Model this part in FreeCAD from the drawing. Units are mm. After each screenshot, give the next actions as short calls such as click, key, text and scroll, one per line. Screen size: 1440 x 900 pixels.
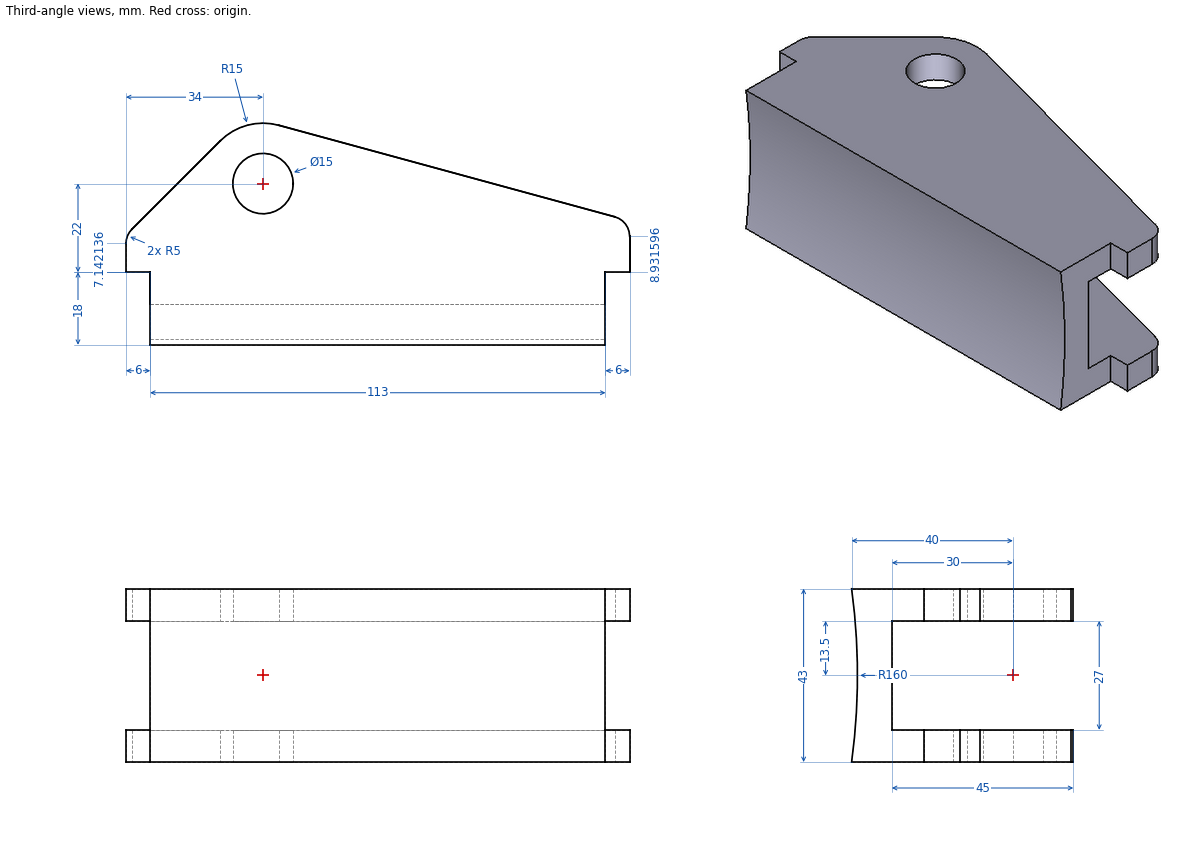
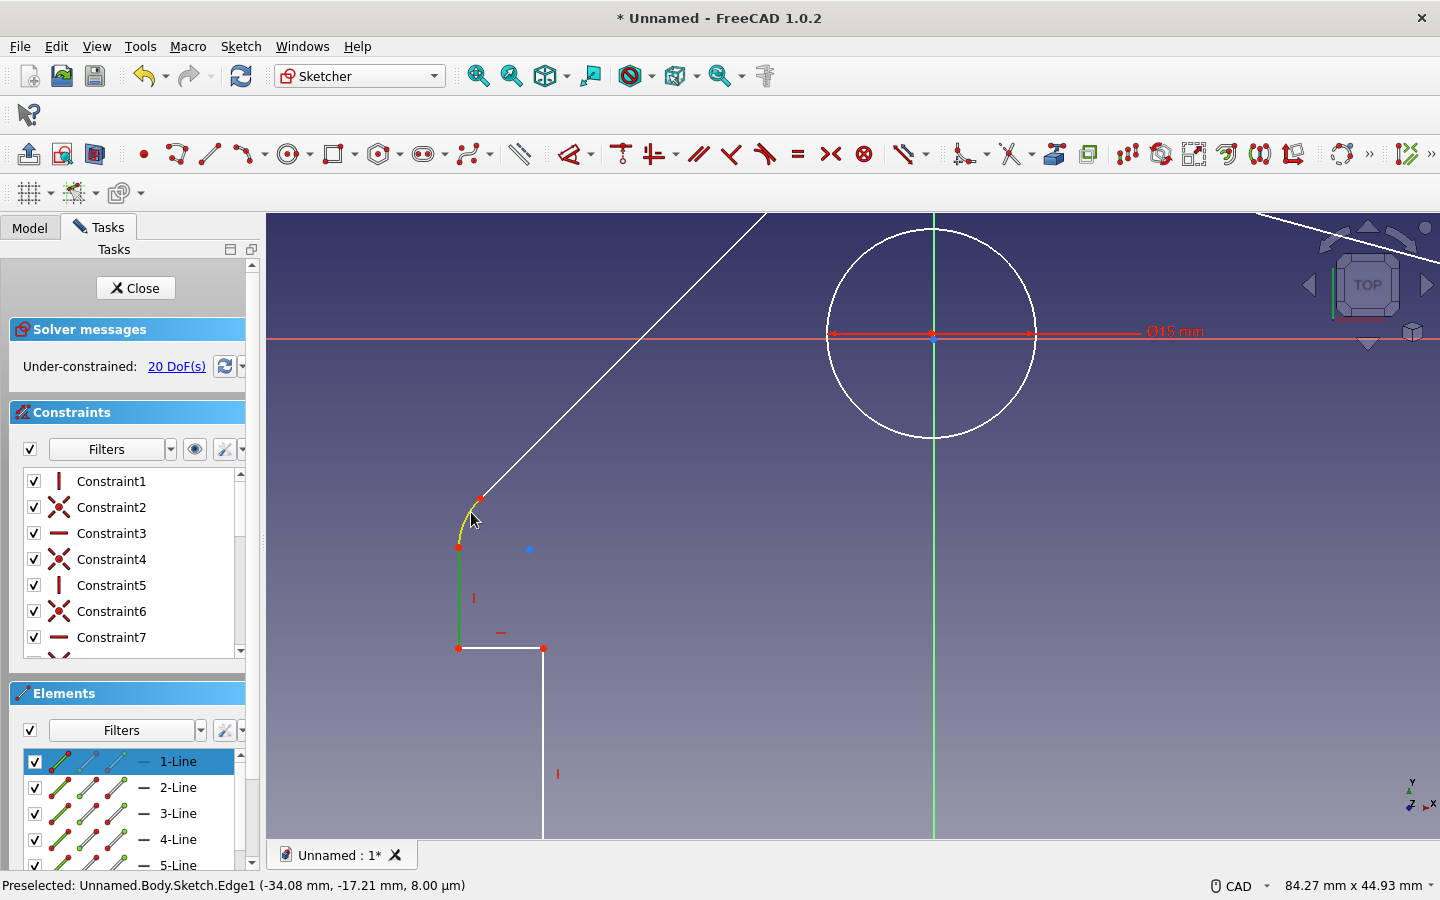
click(470, 511)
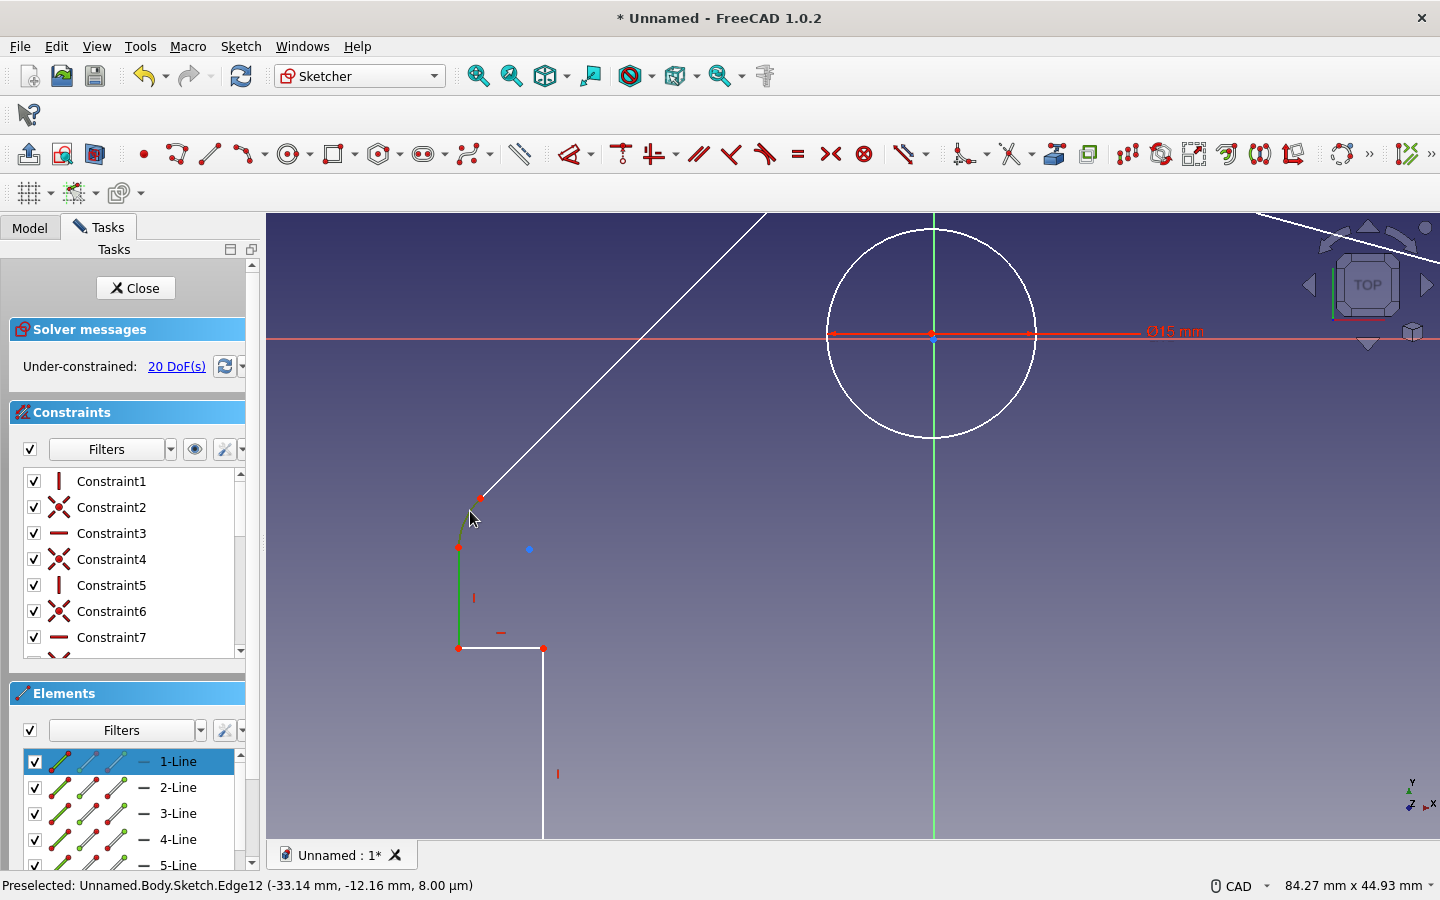
click(765, 154)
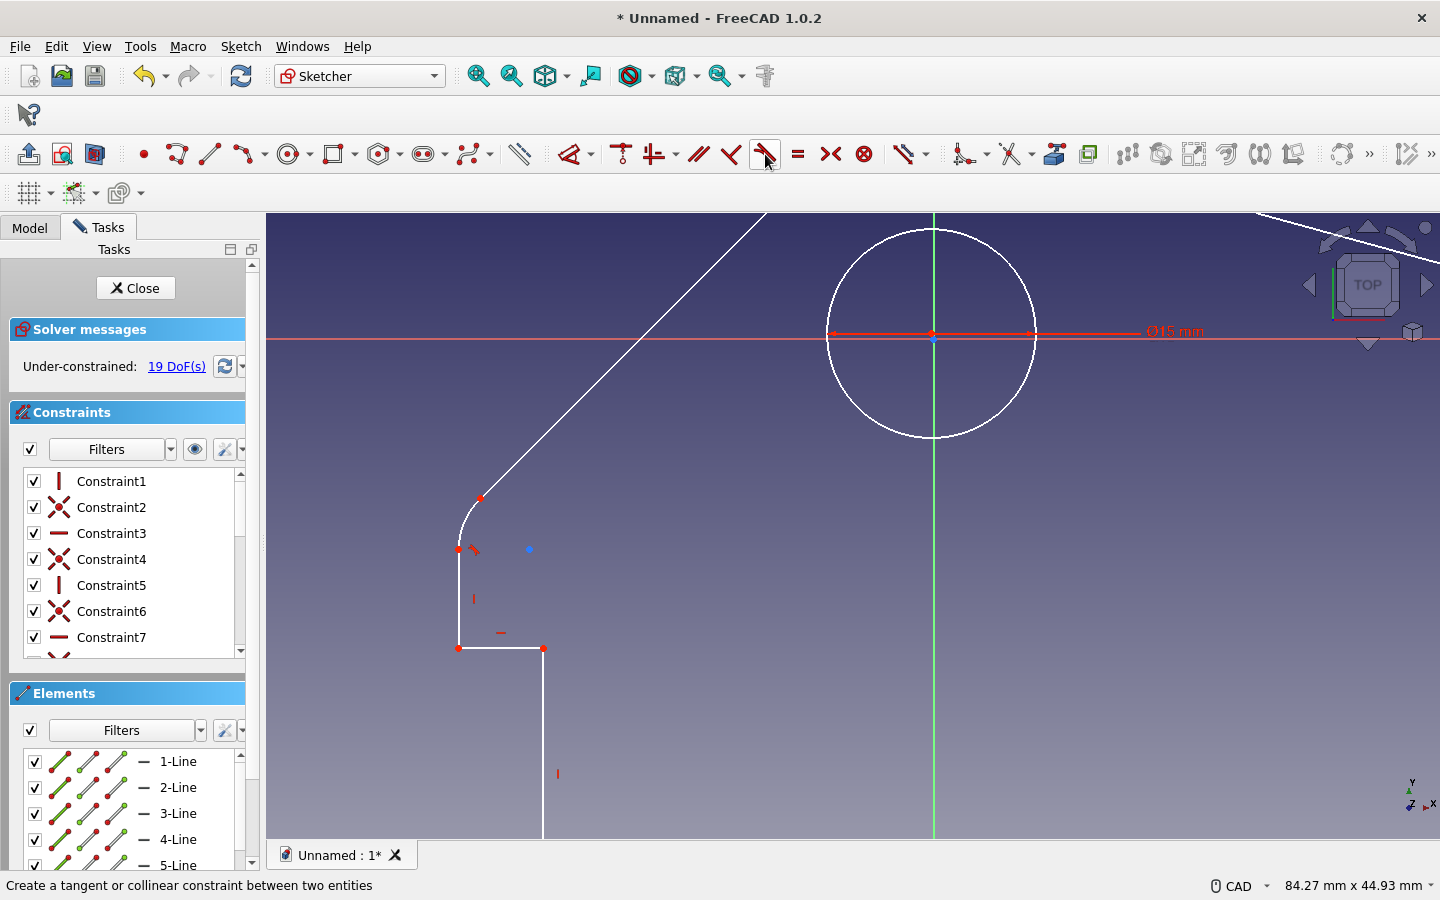
scroll(467, 531, down, 5)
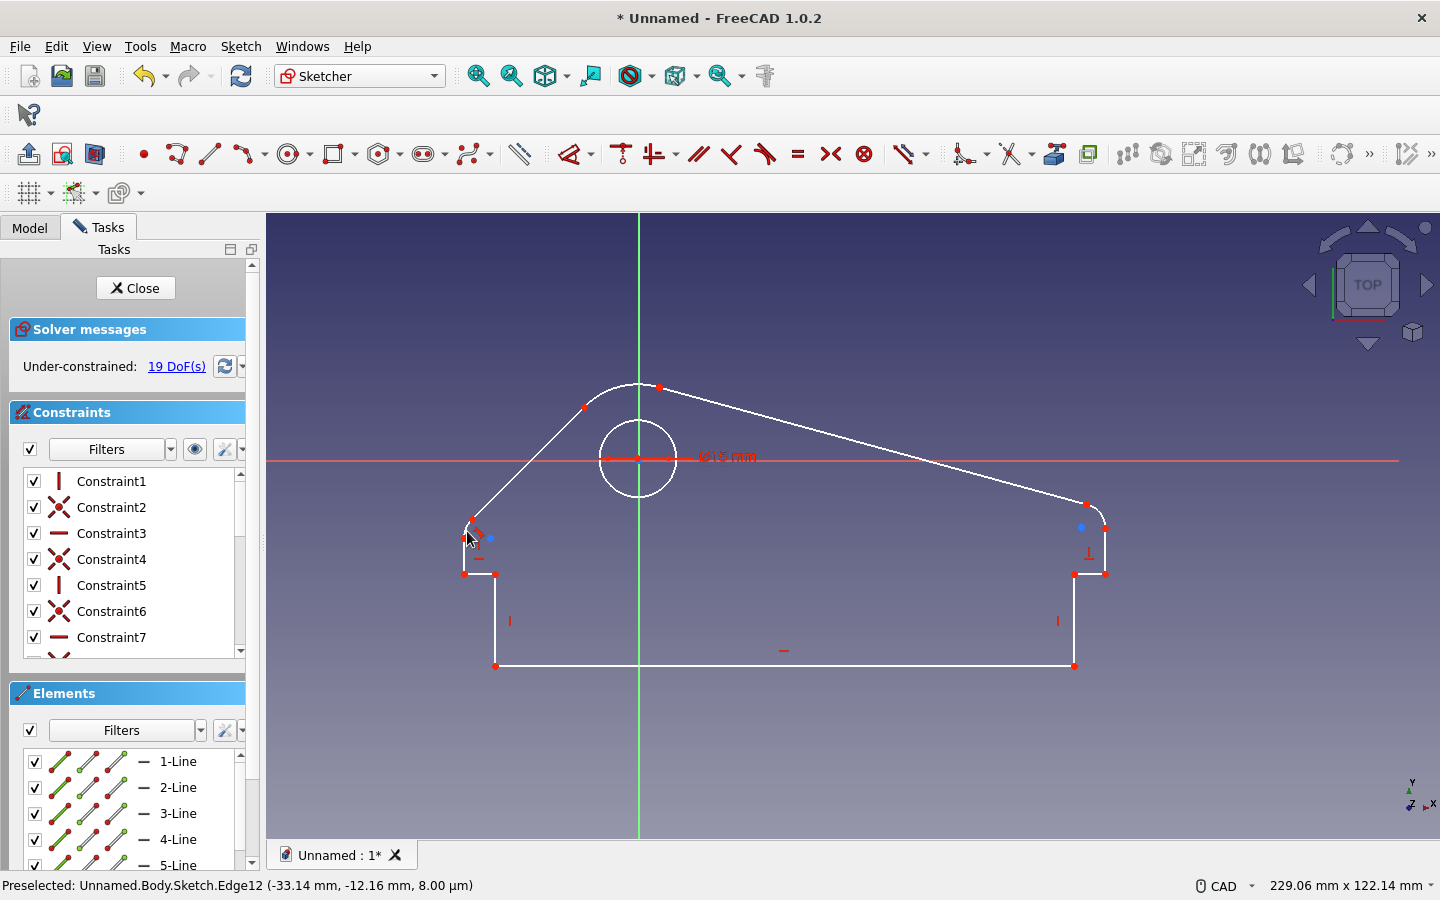
click(1105, 561)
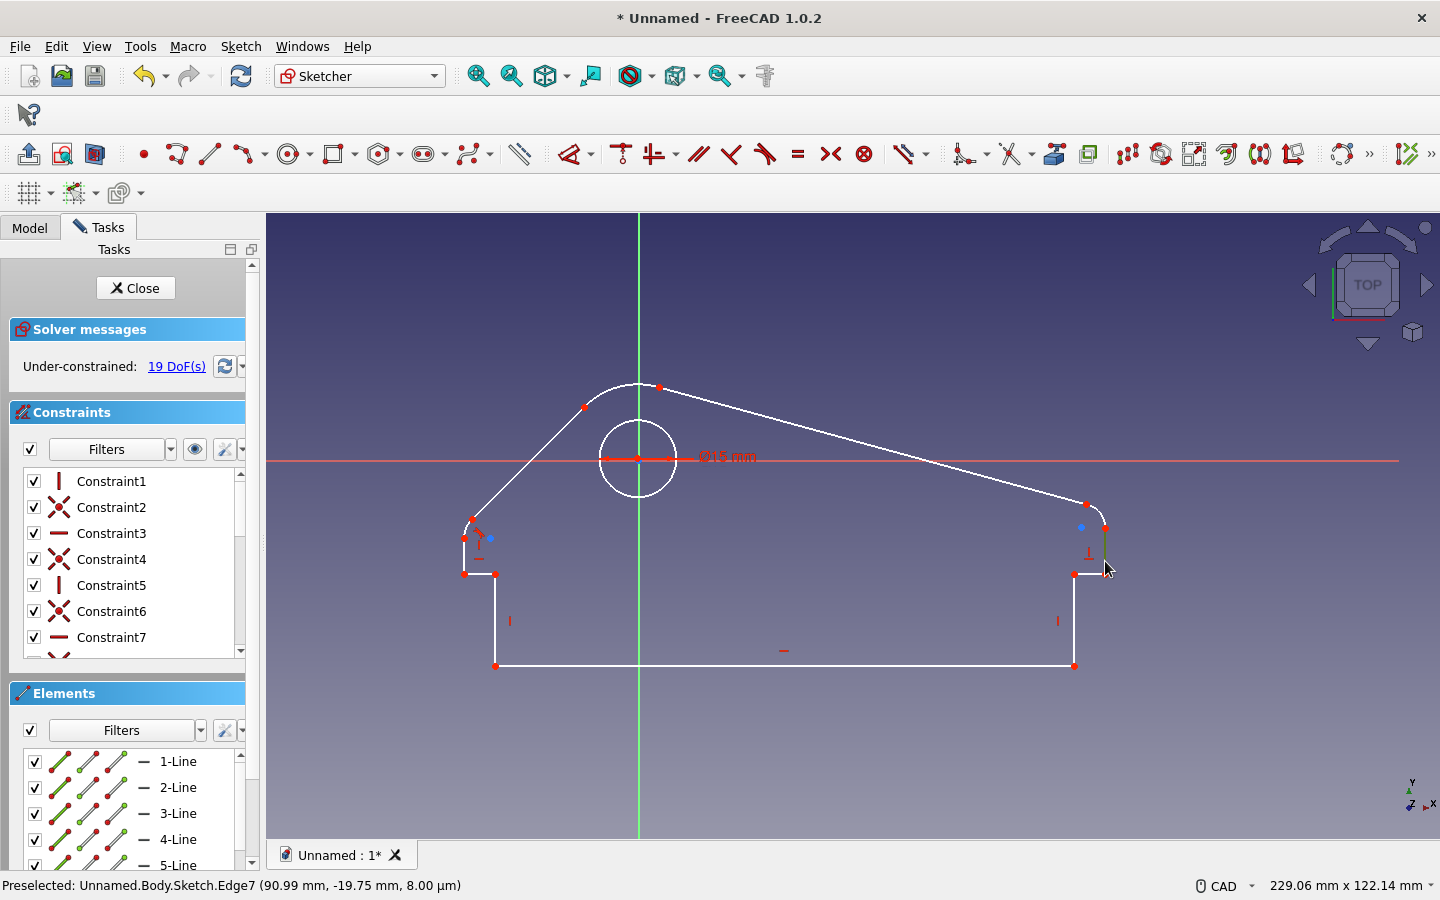
scroll(1103, 519, up, 2)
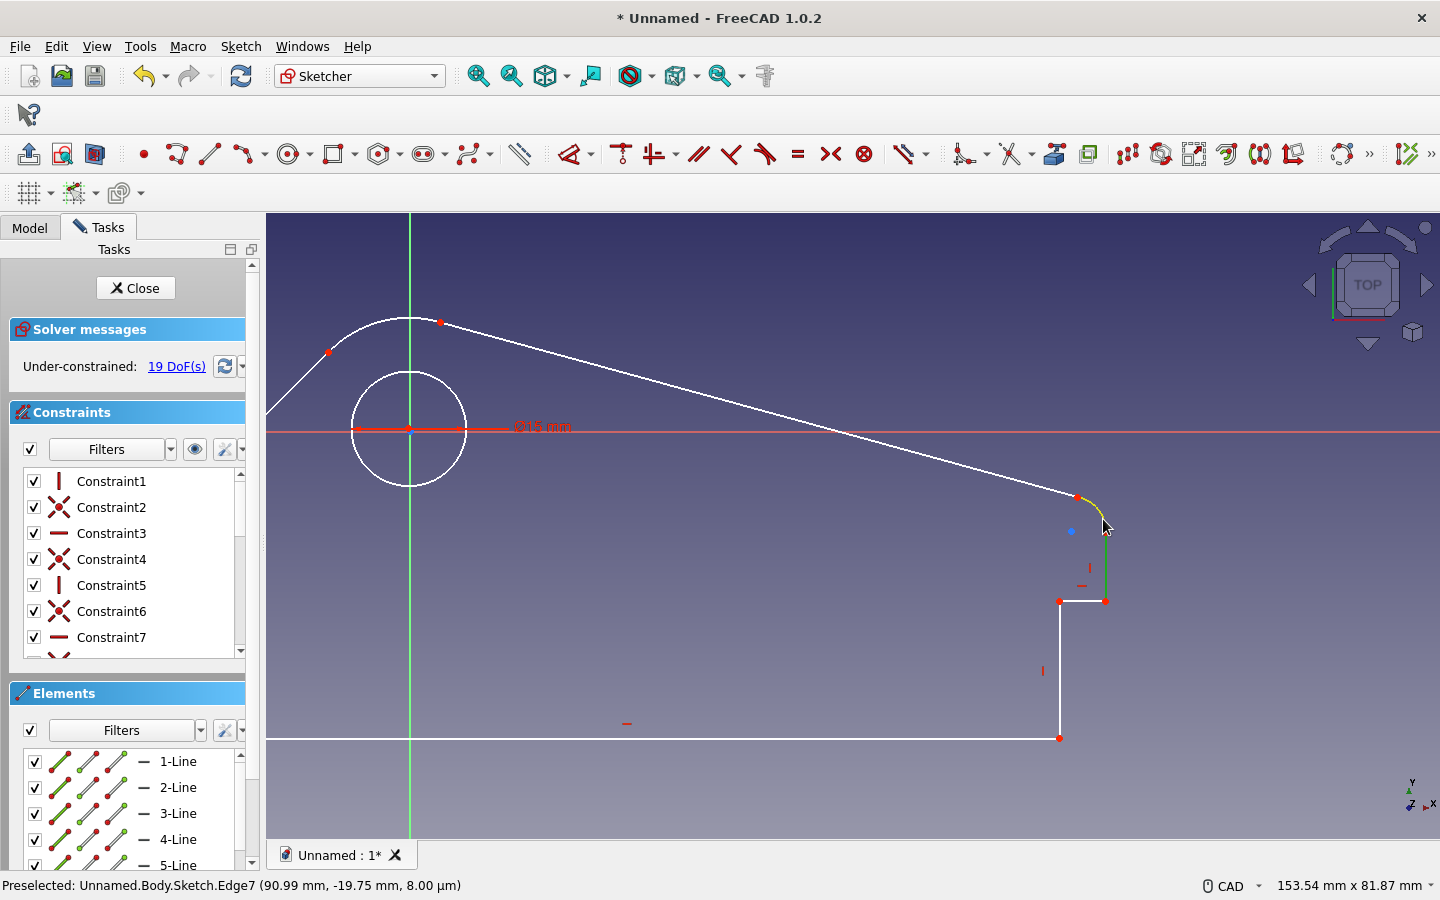
click(1103, 518)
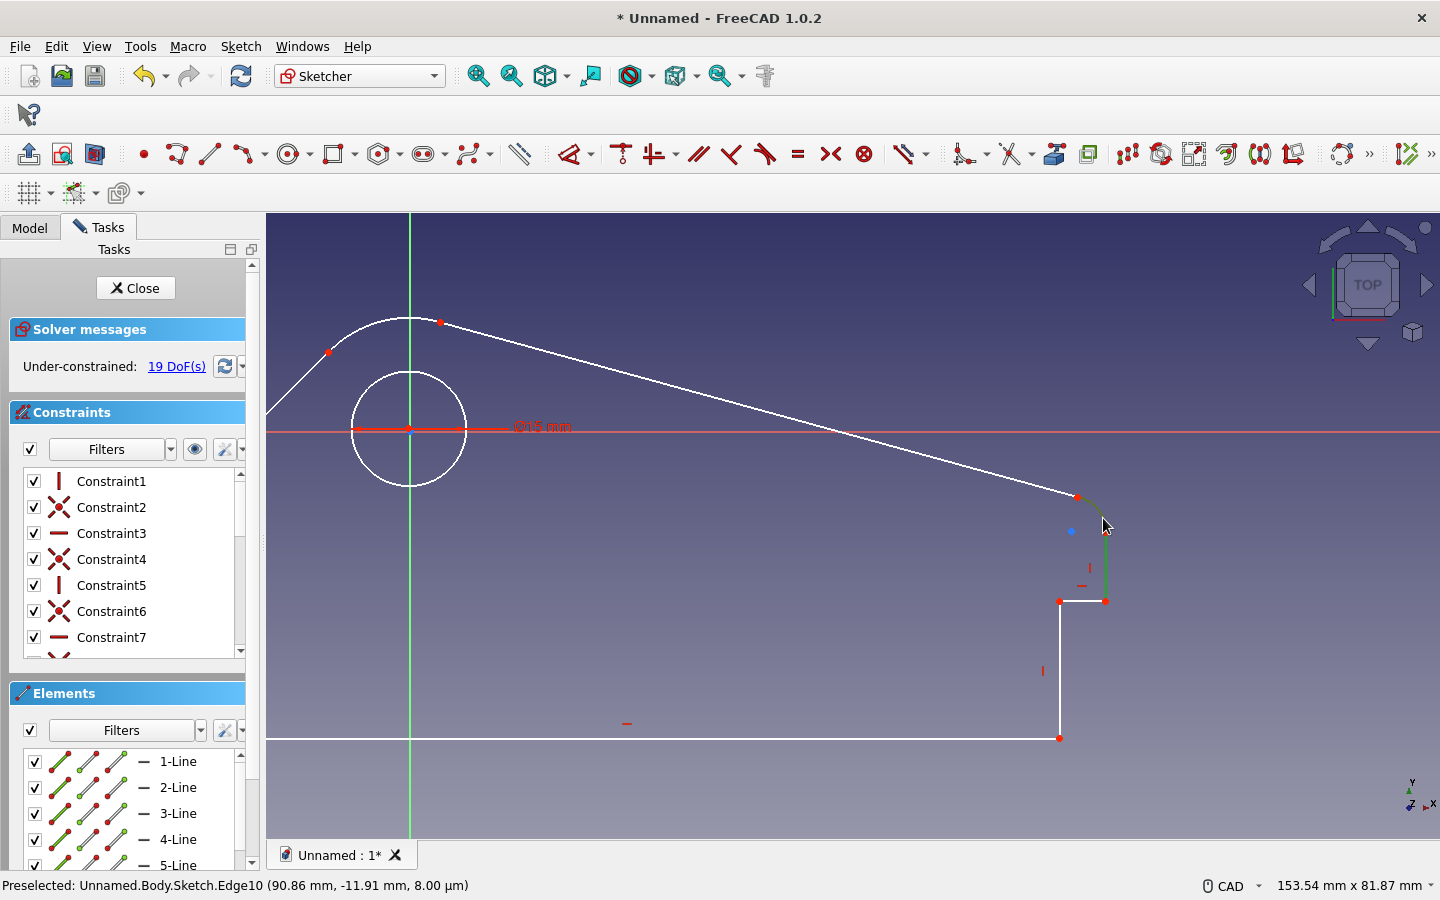
click(765, 154)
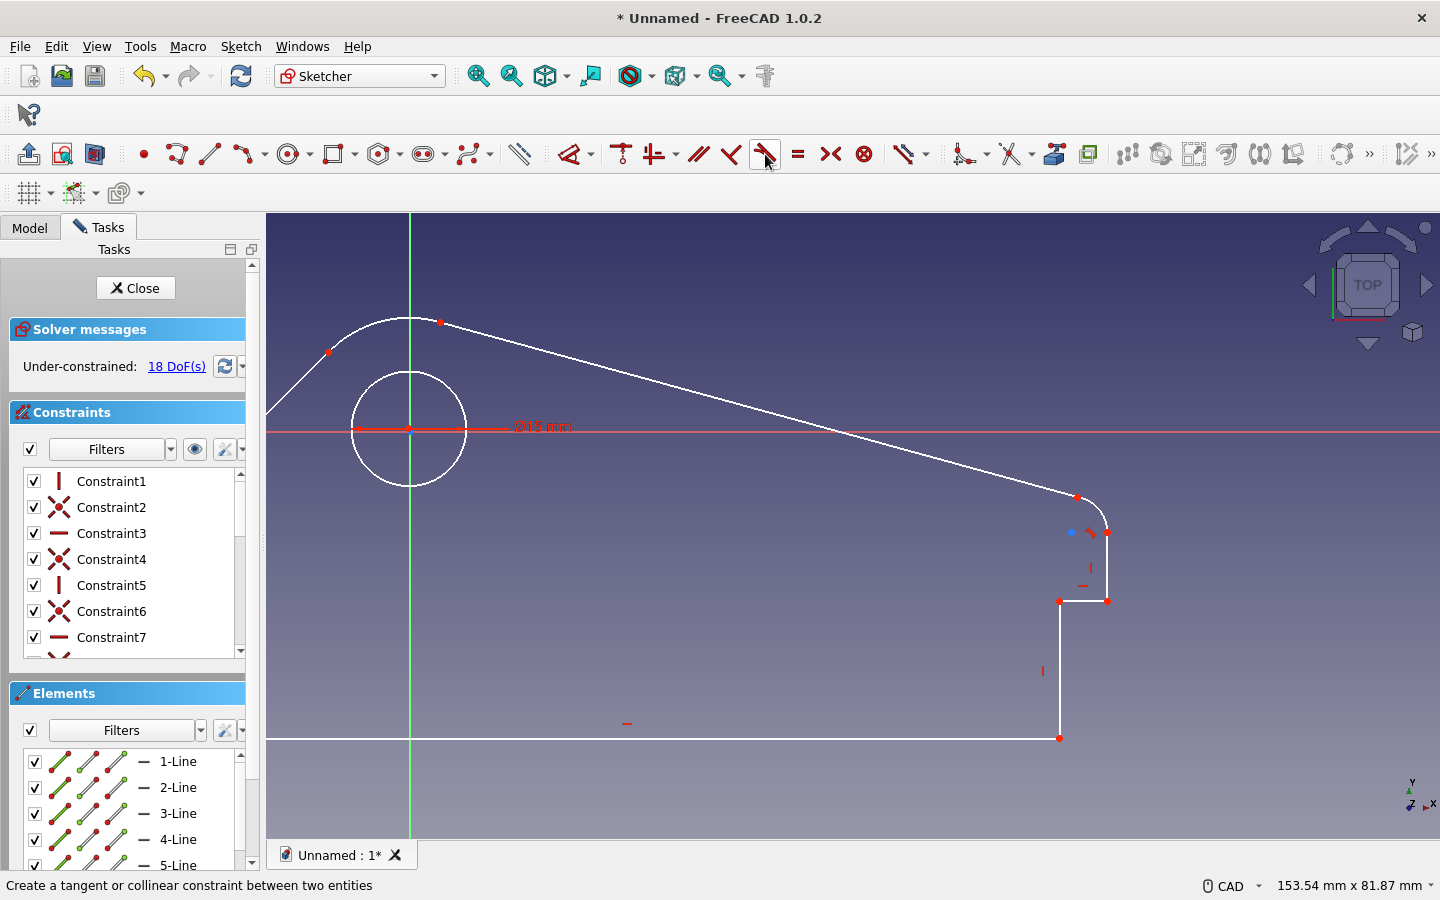
click(886, 445)